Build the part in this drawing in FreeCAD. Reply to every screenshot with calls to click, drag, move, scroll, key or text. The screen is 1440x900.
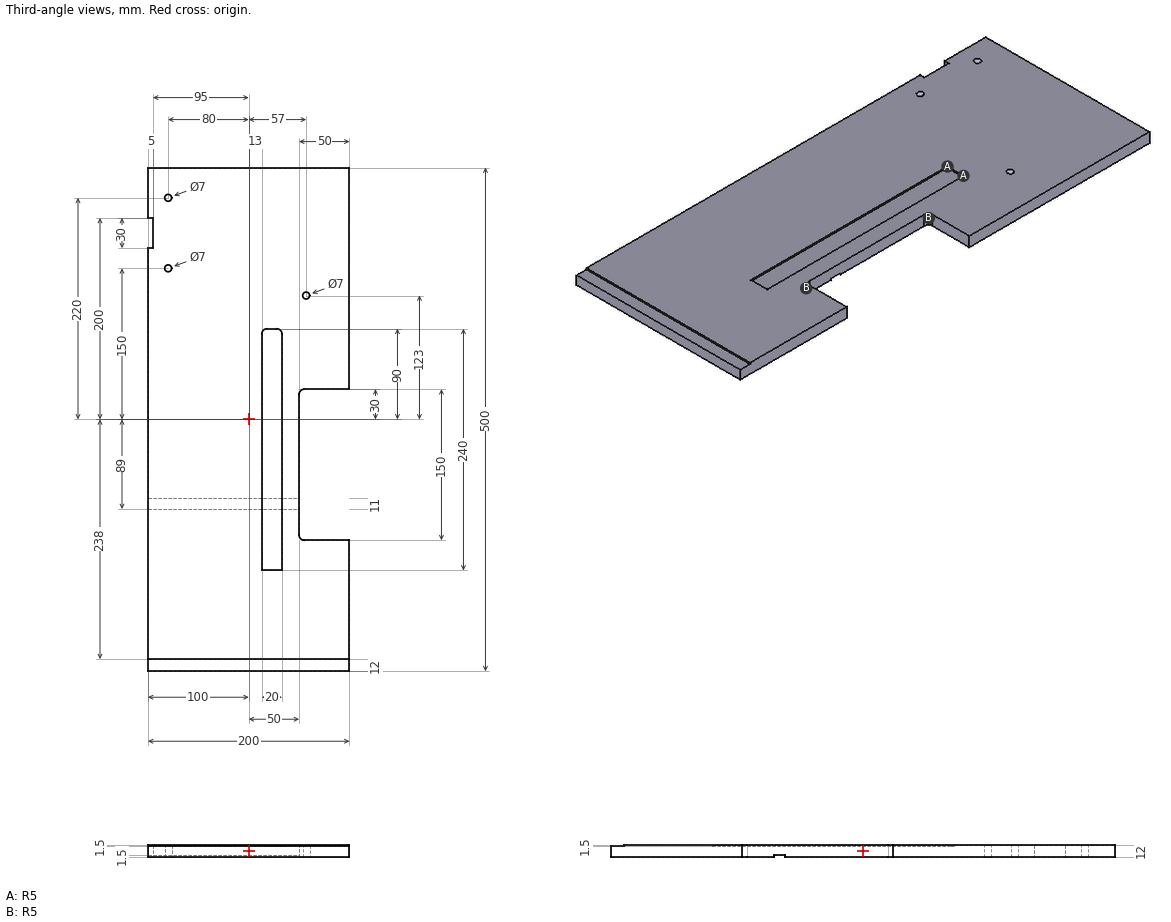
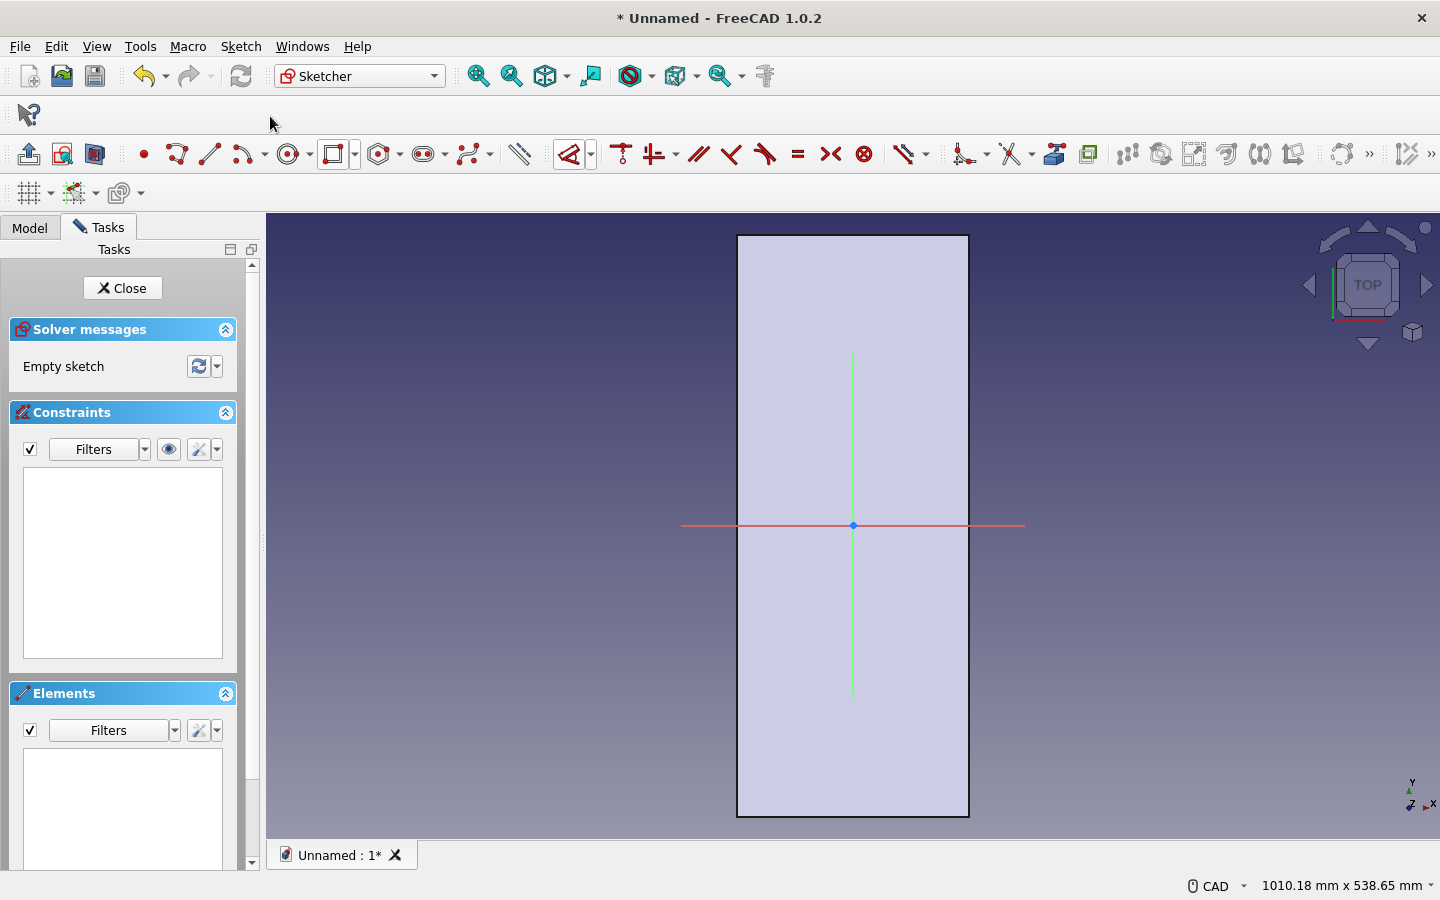
scroll(735, 290, up, 12)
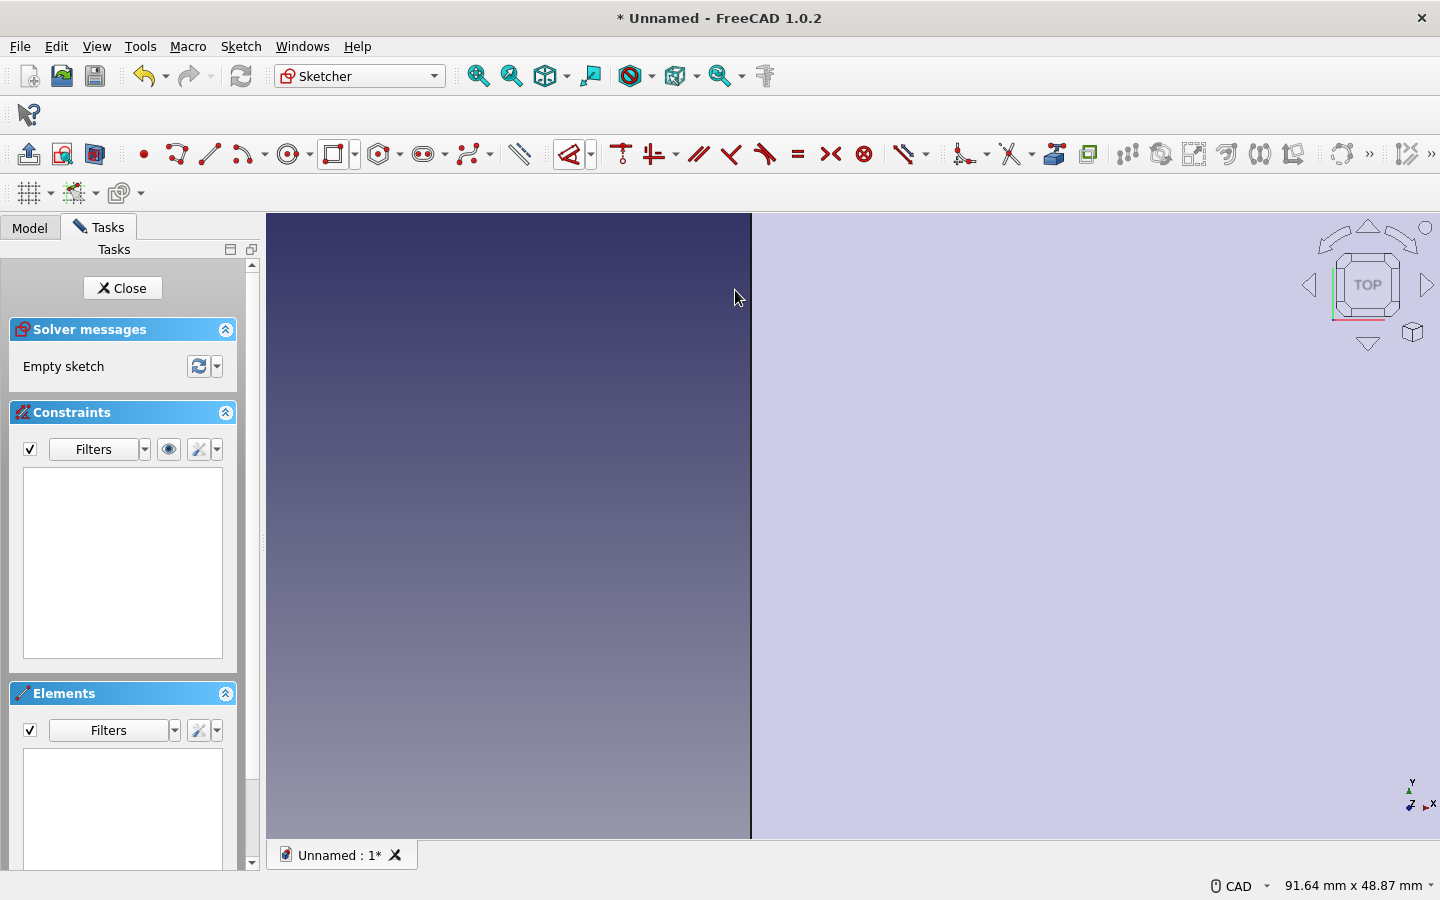
key(g)
key(r)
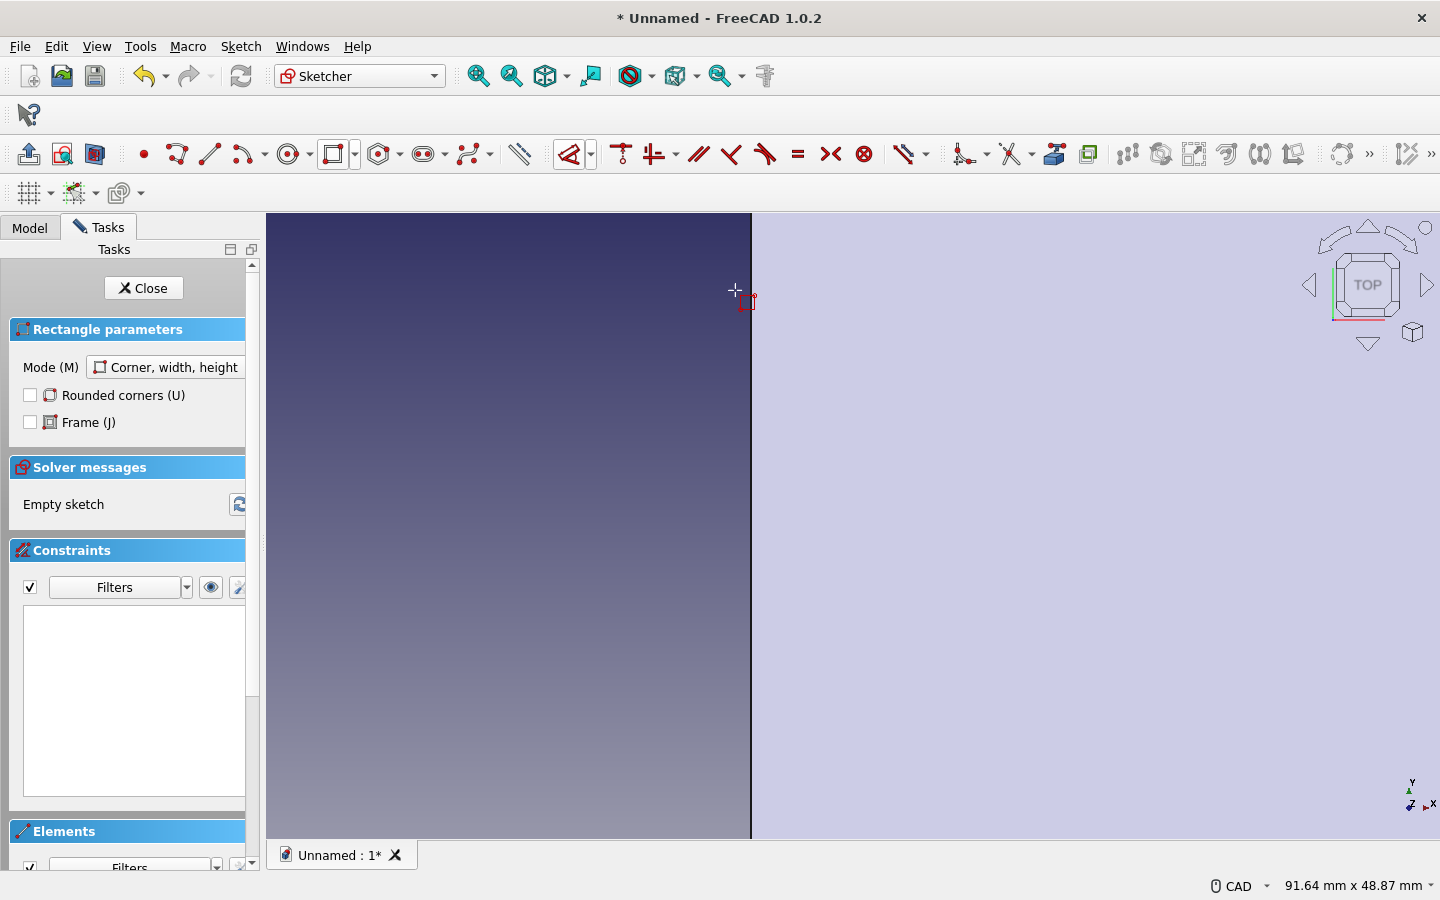
click(751, 328)
move(815, 712)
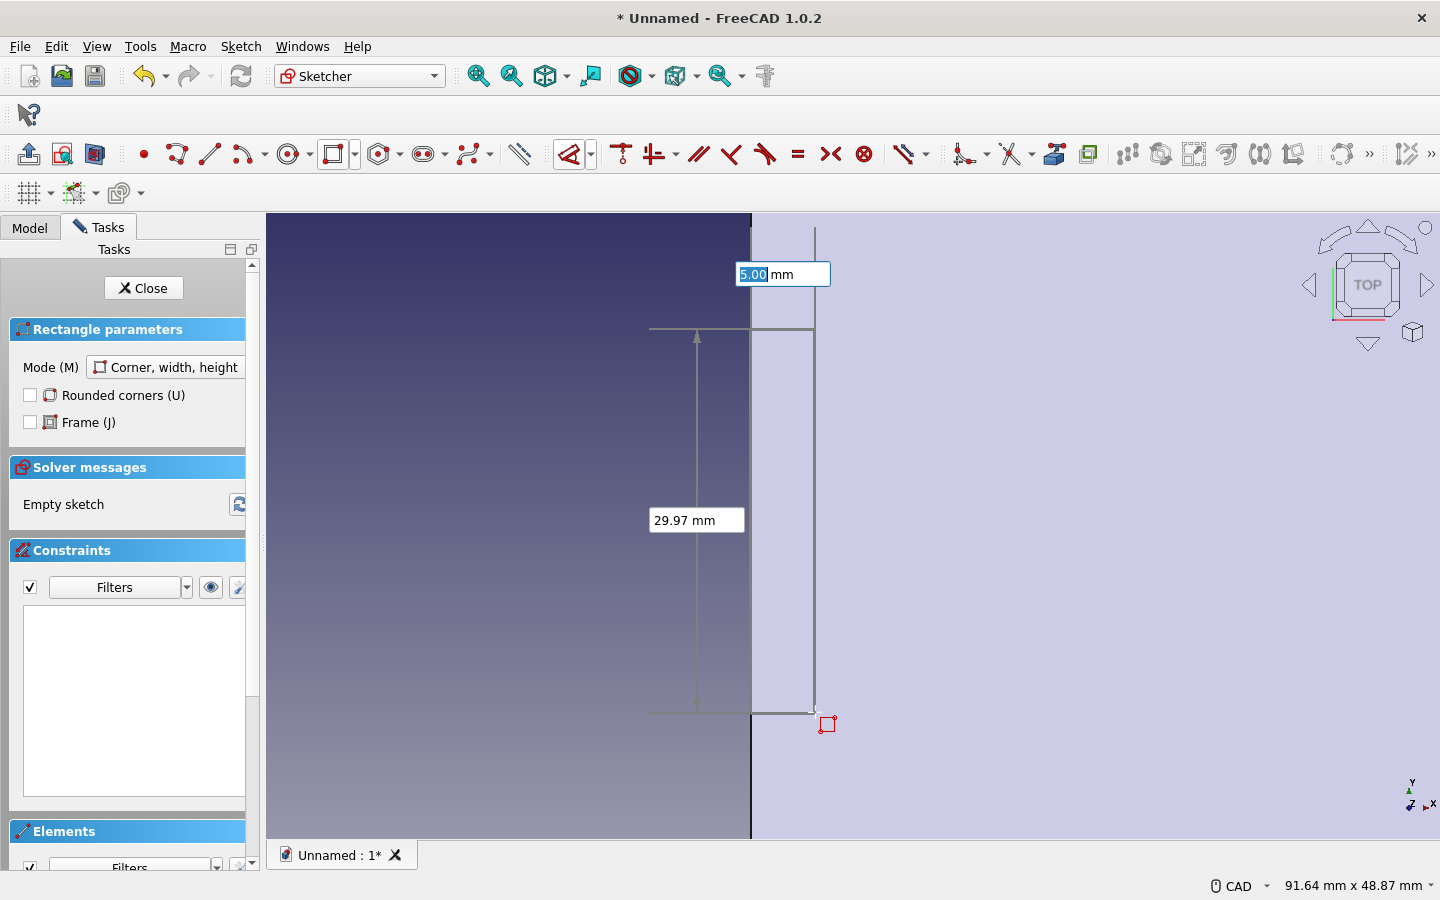
text(5)
key(Tab)
text(30)
key(Return)
key(Escape)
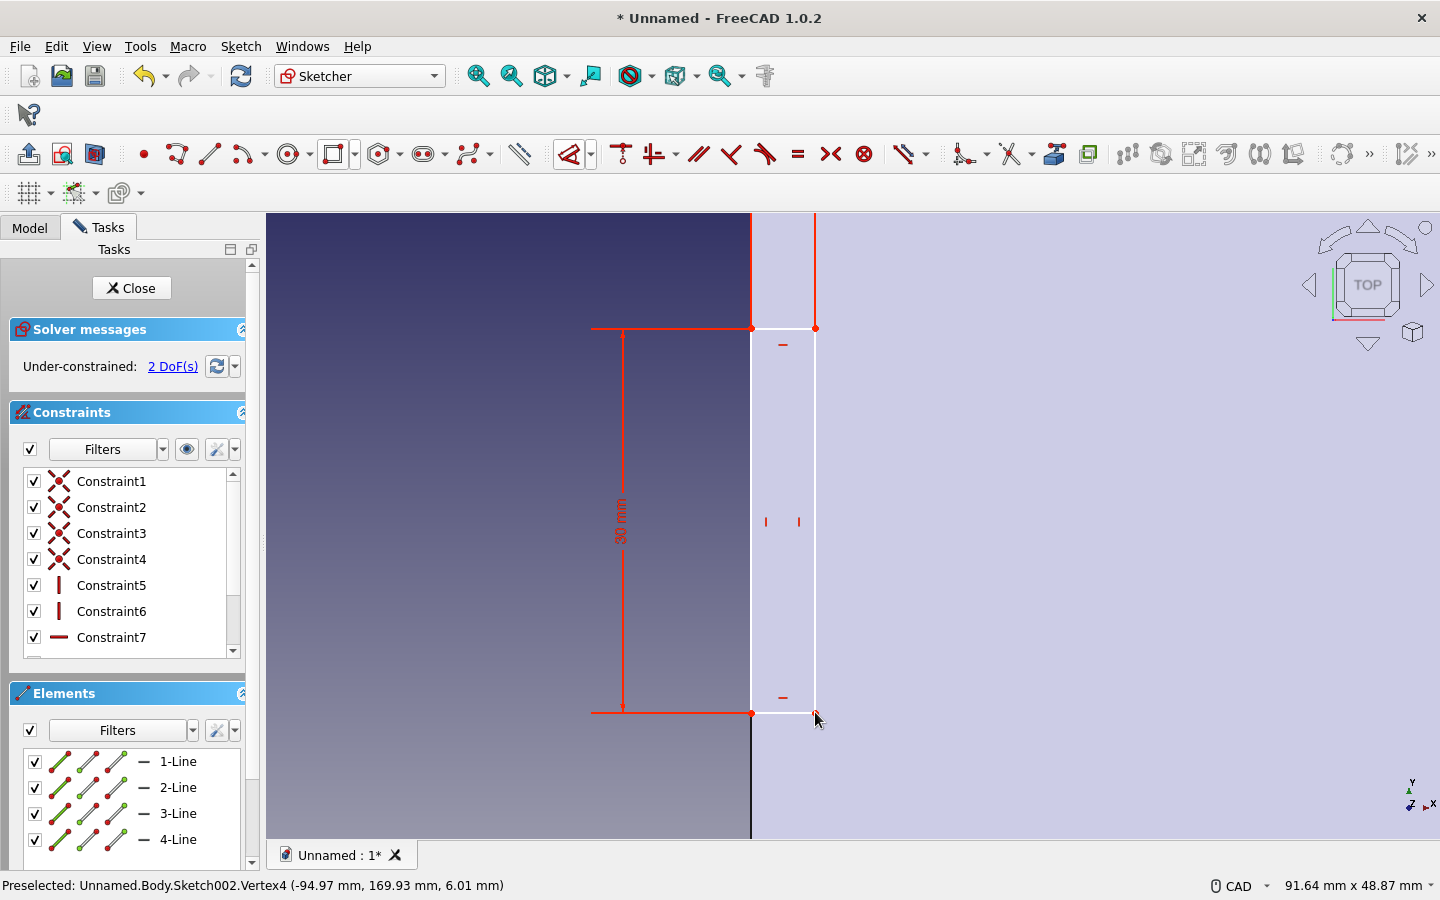
click(568, 154)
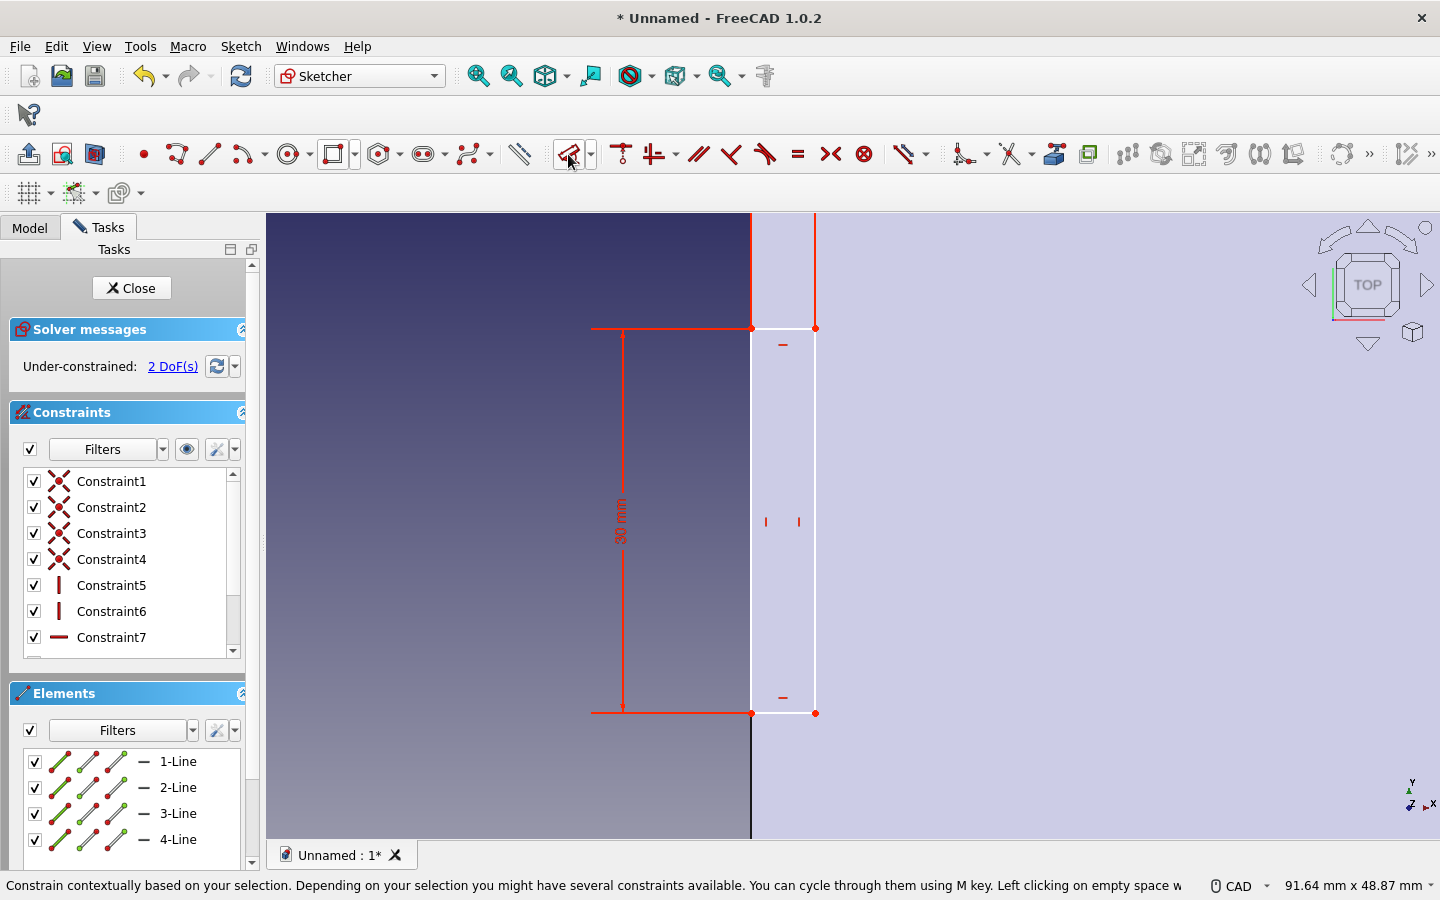
click(815, 713)
click(1045, 679)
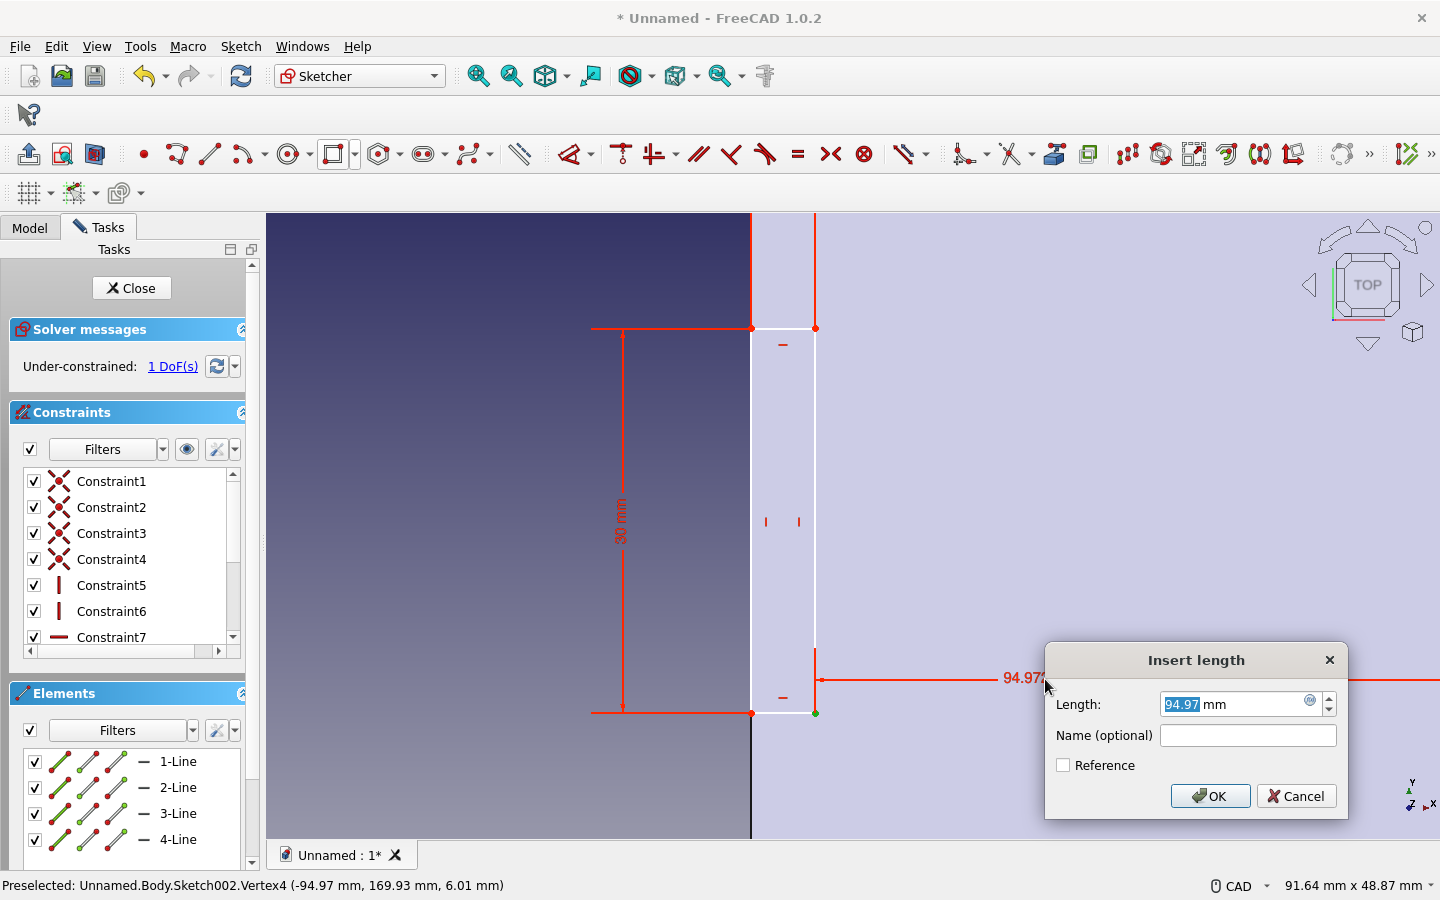
text(95)
key(Return)